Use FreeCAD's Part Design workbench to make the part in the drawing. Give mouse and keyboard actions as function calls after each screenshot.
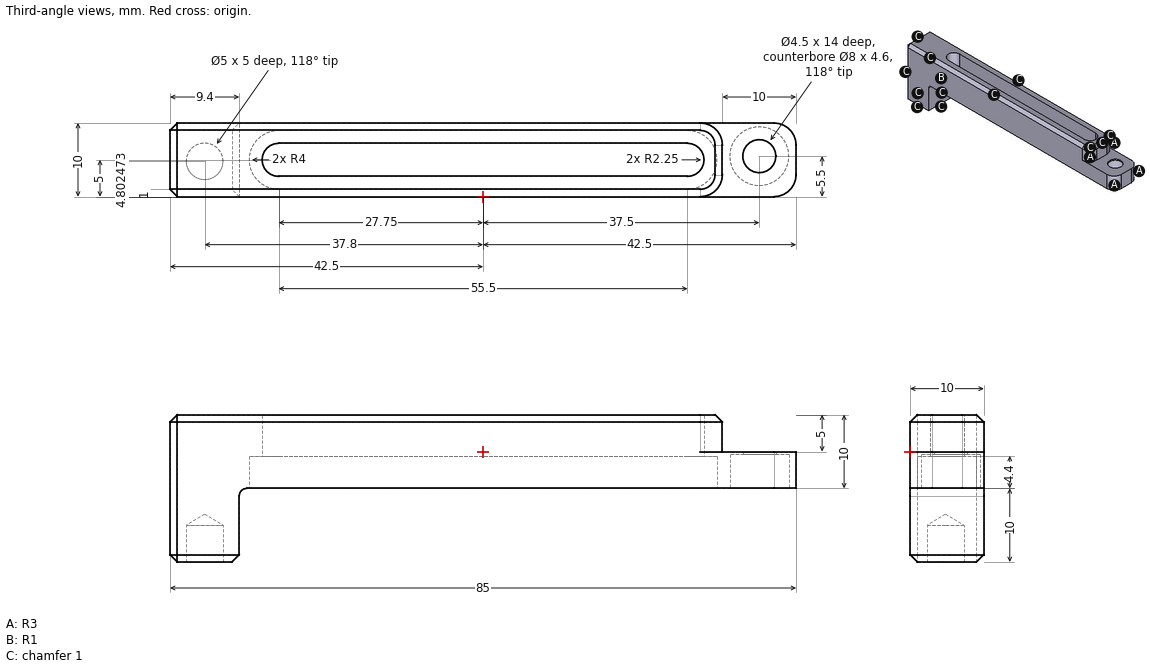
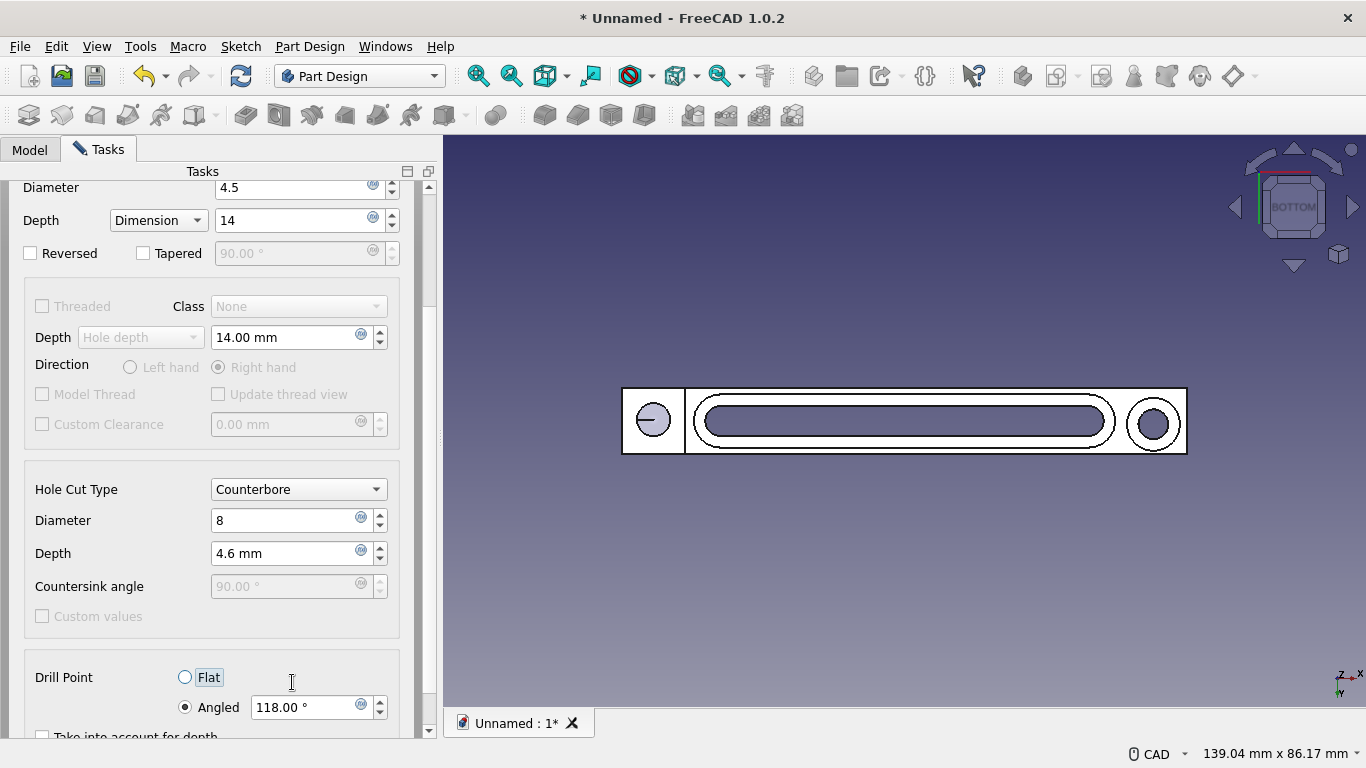
scroll(429, 460, up, 4)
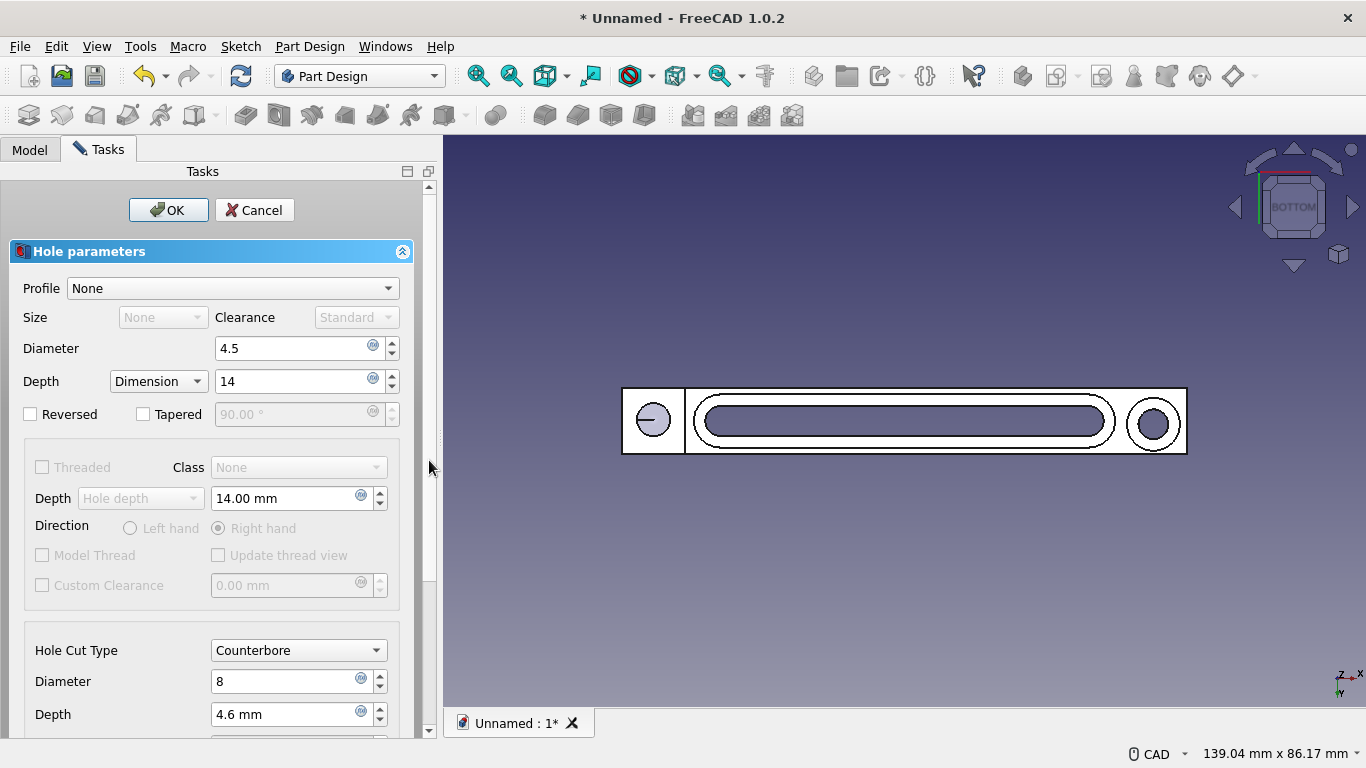
click(169, 210)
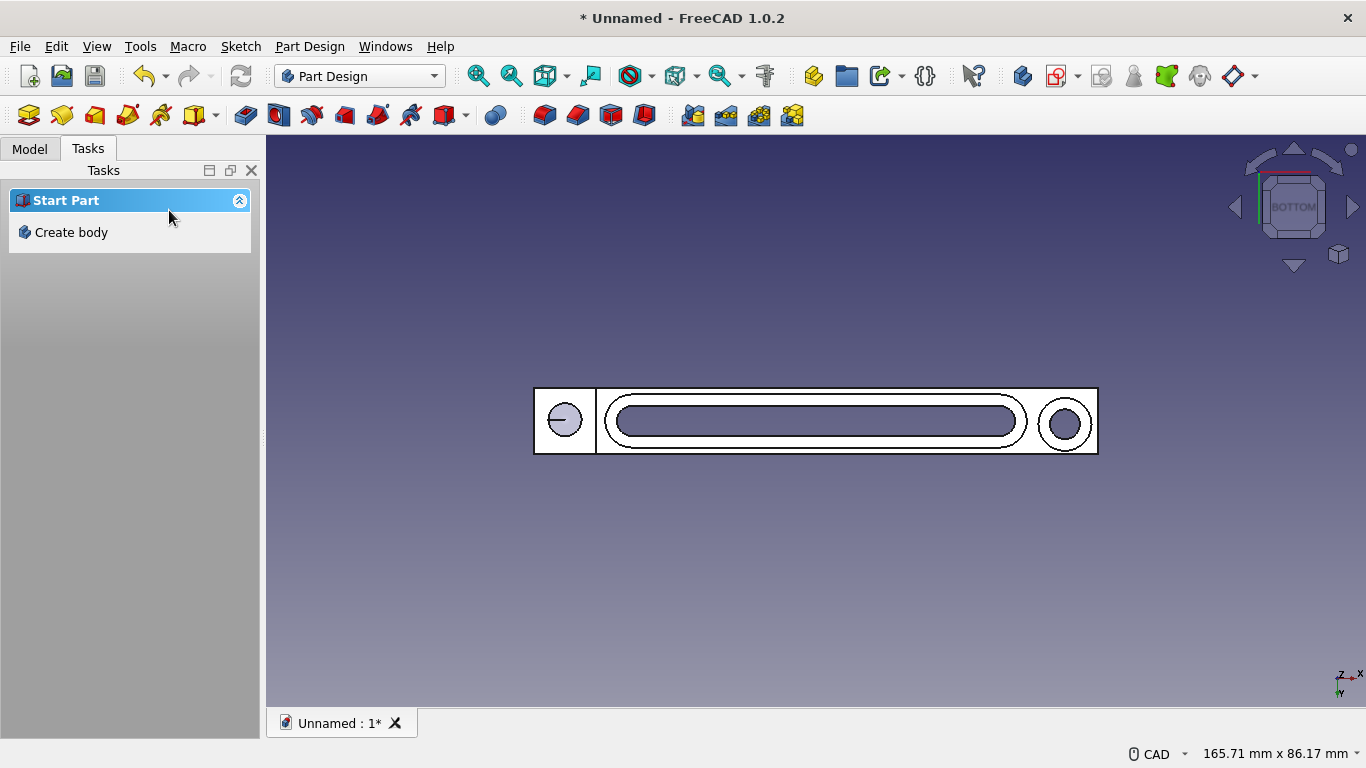
key(0)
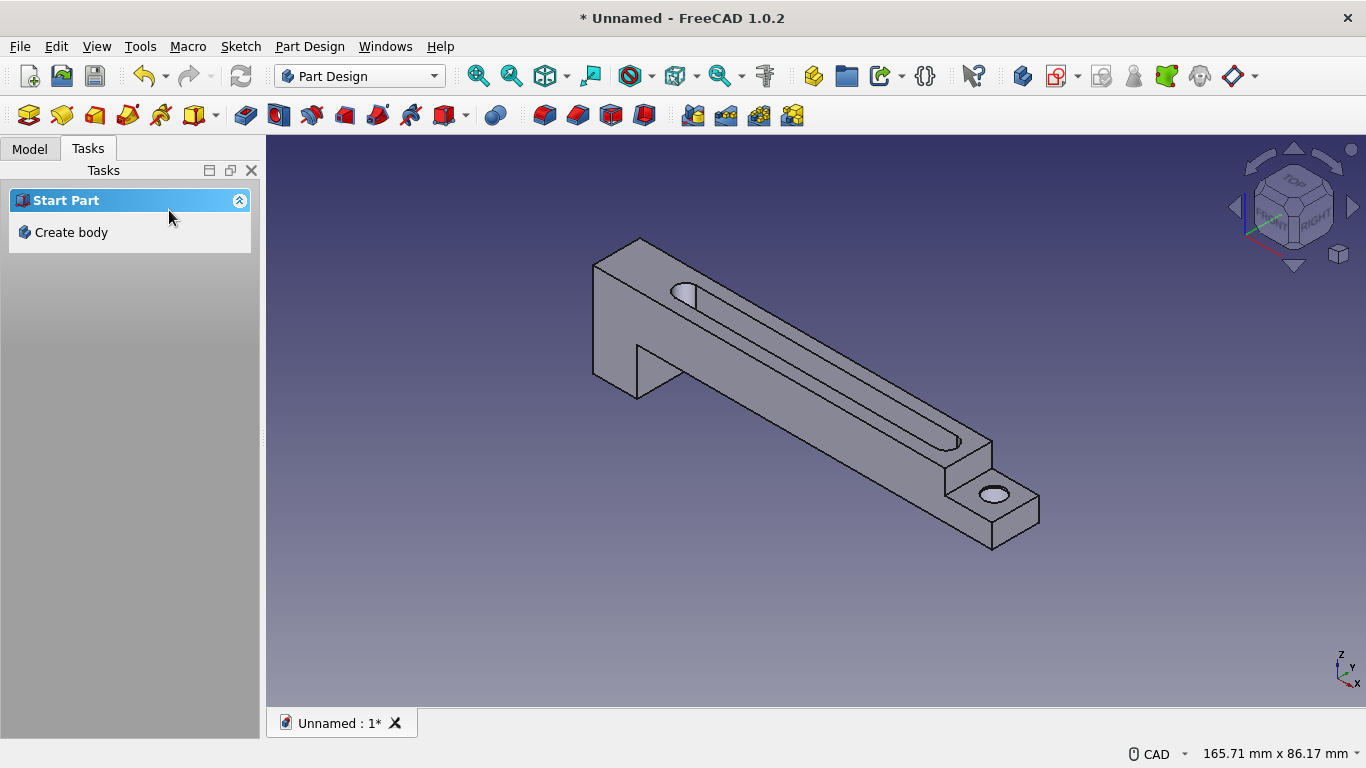
click(992, 535)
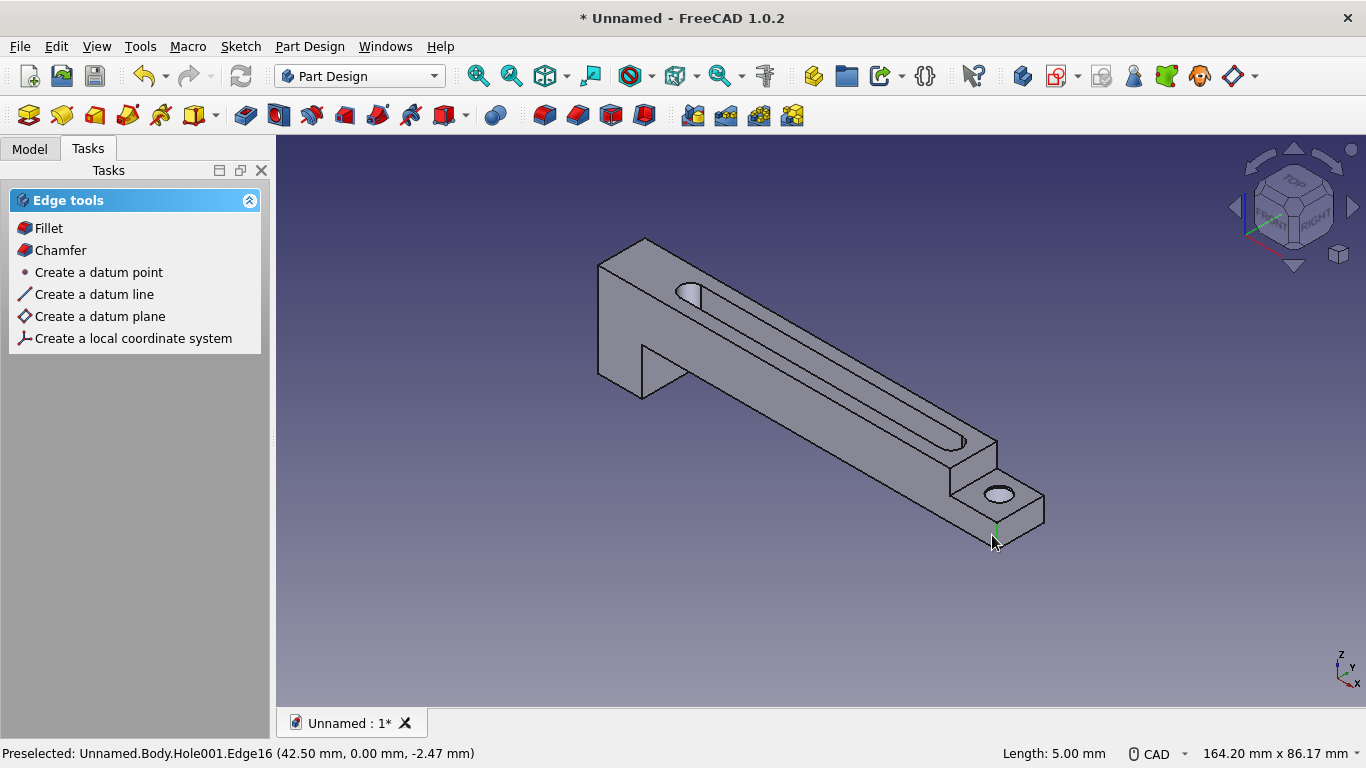
click(950, 481, ctrl)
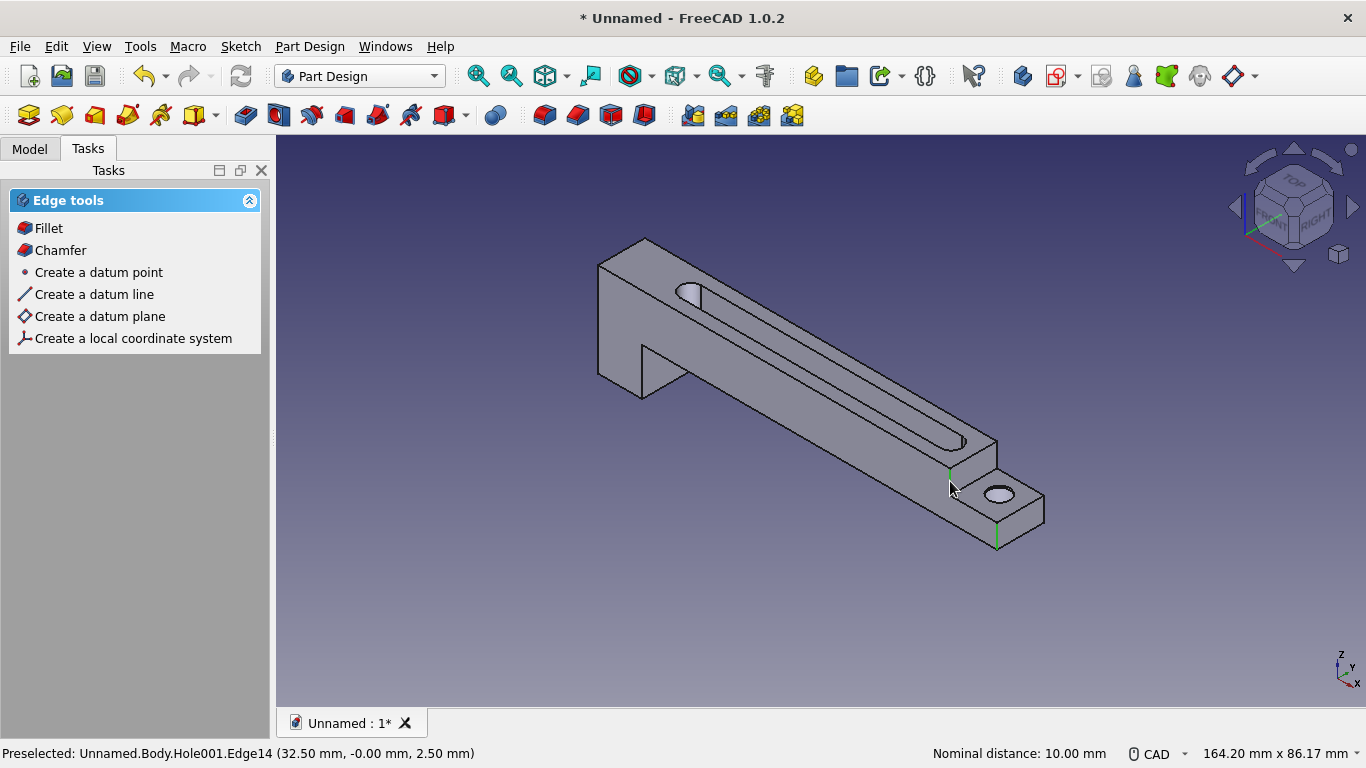
key(2)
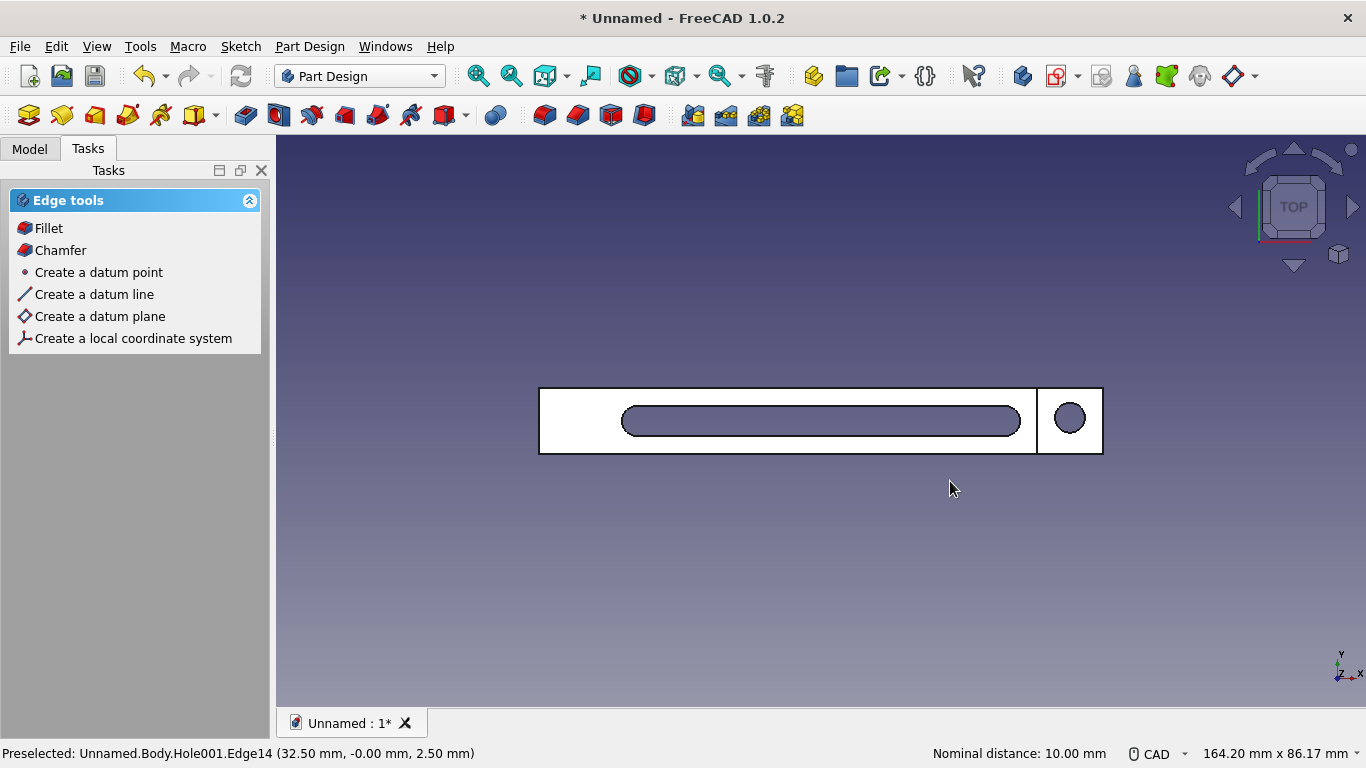
key(1)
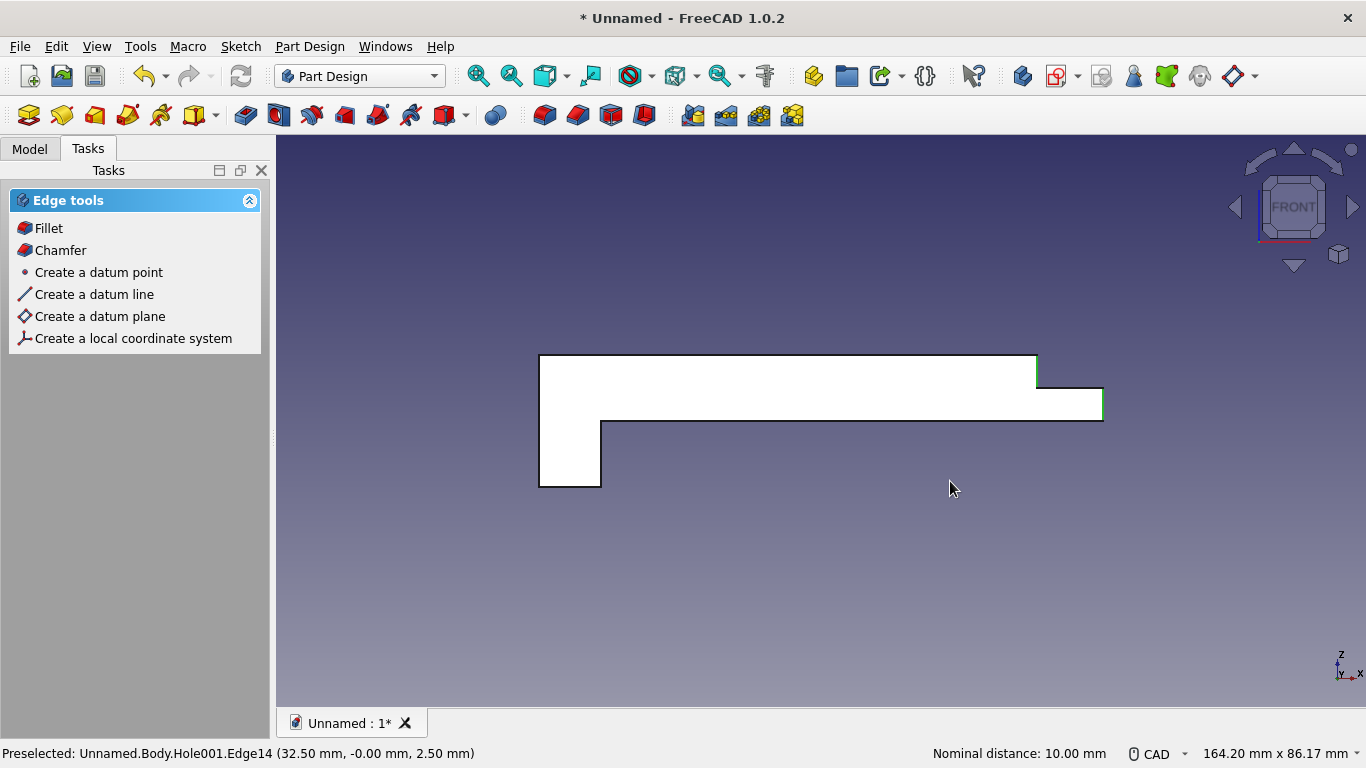
key(3)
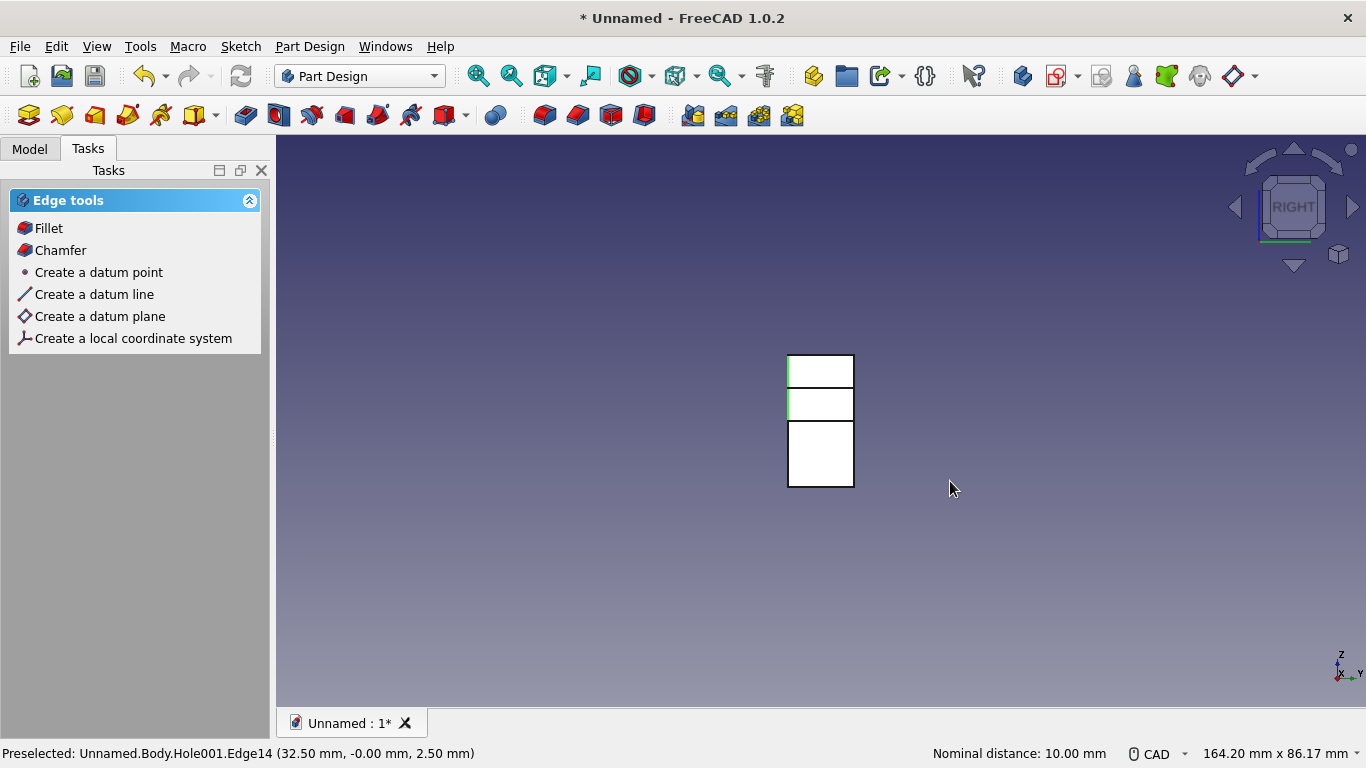
key(v)
key(f)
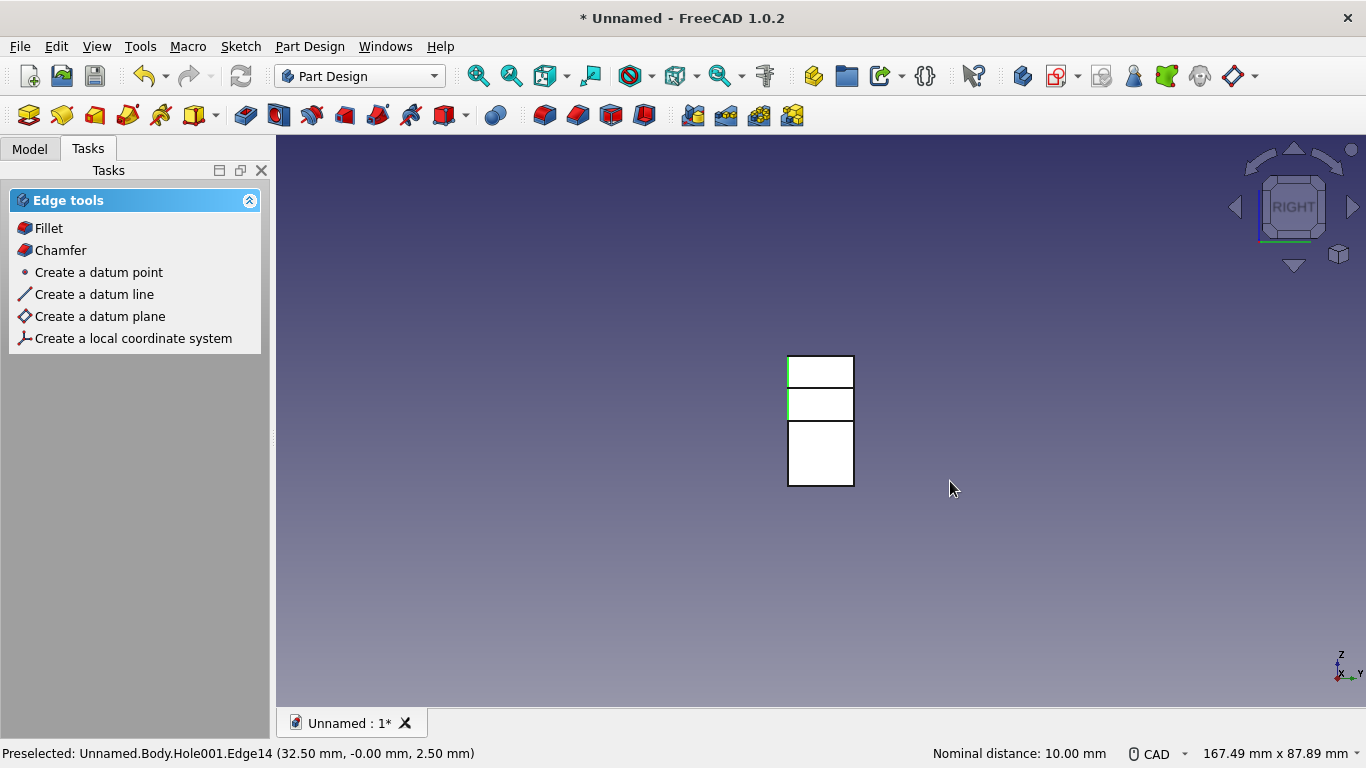
click(854, 404, ctrl)